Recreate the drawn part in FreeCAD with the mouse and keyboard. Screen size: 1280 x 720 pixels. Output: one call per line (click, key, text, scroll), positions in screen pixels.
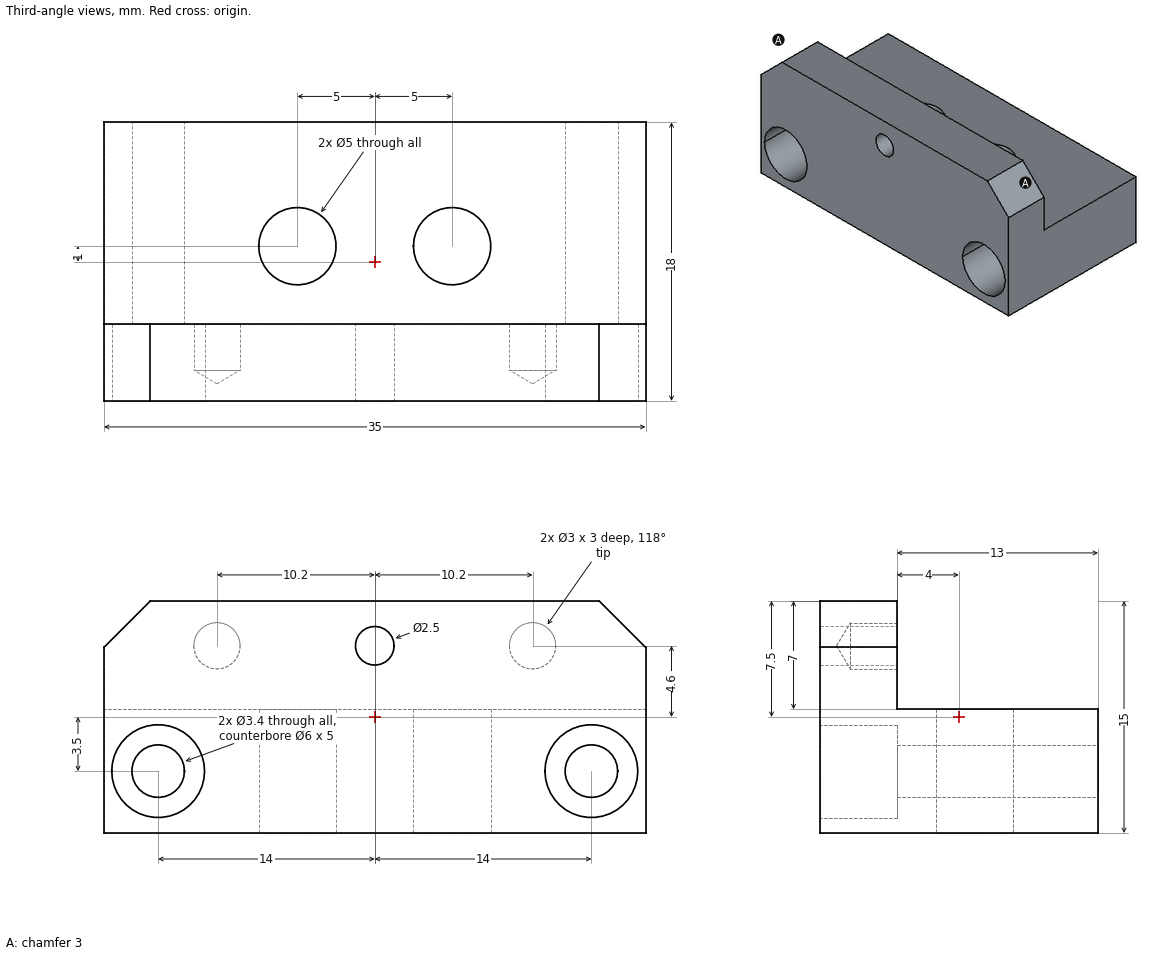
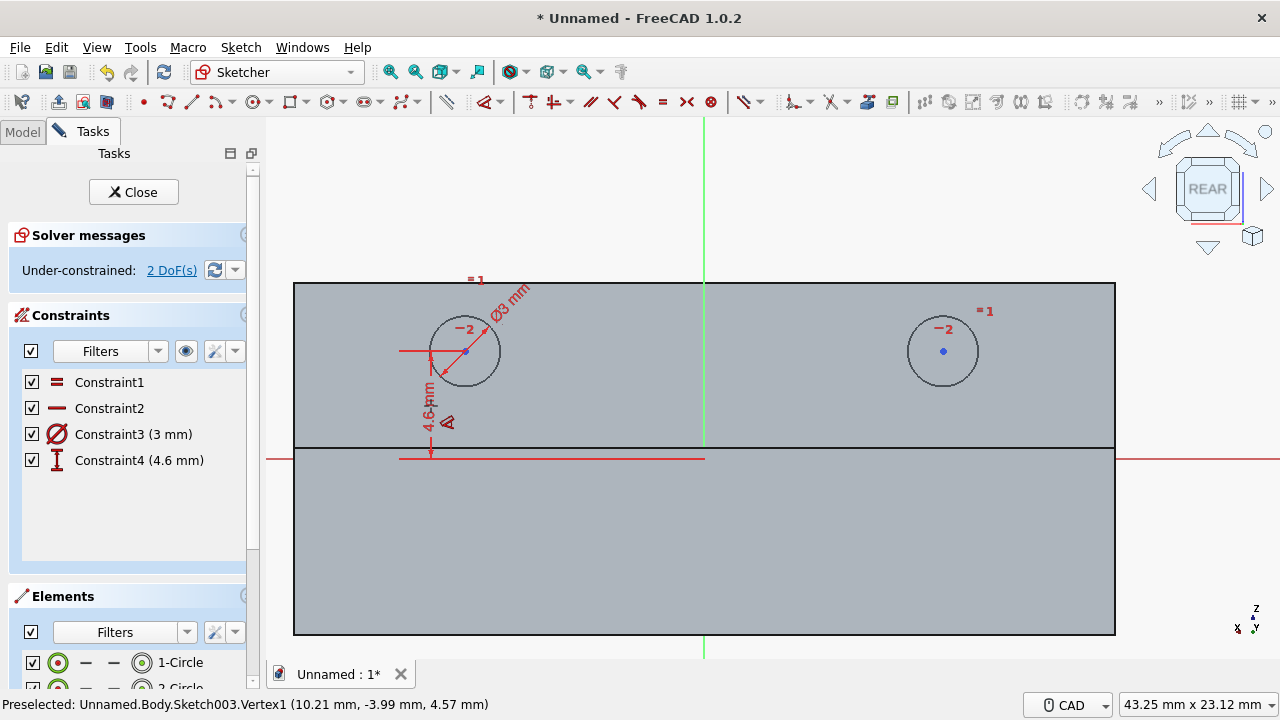
click(465, 351)
click(585, 493)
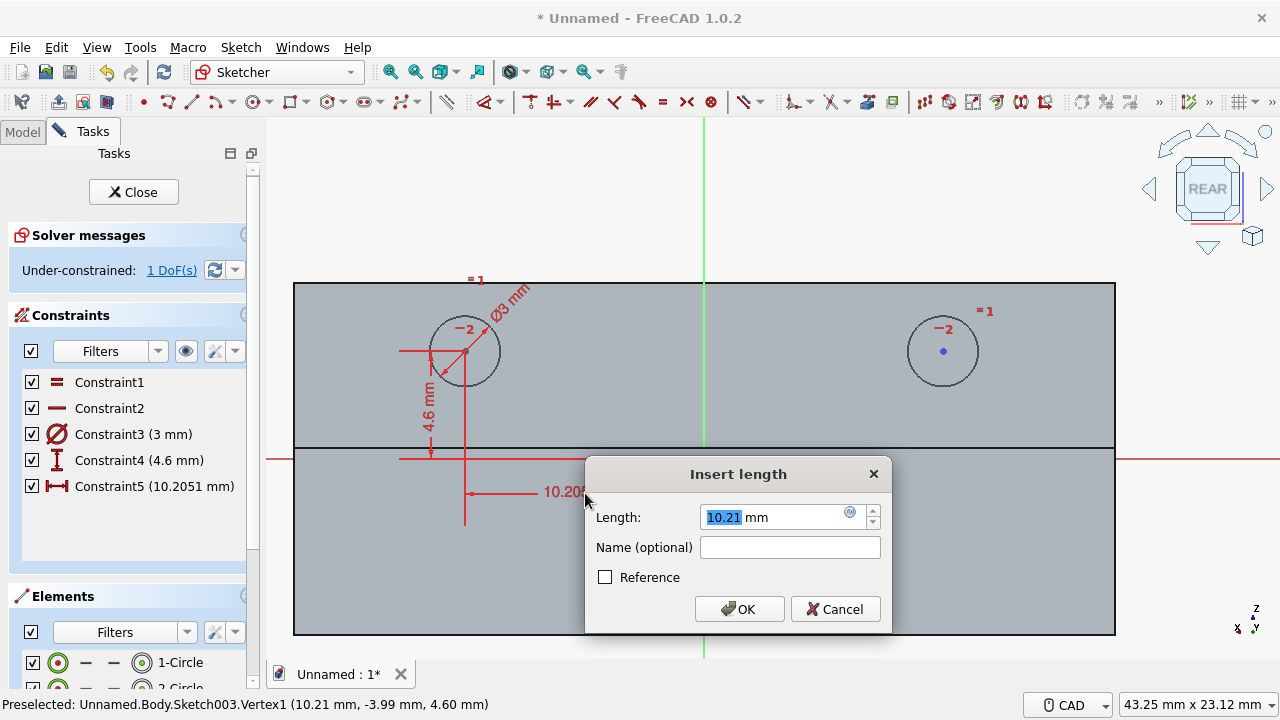
text(10.2)
key(Return)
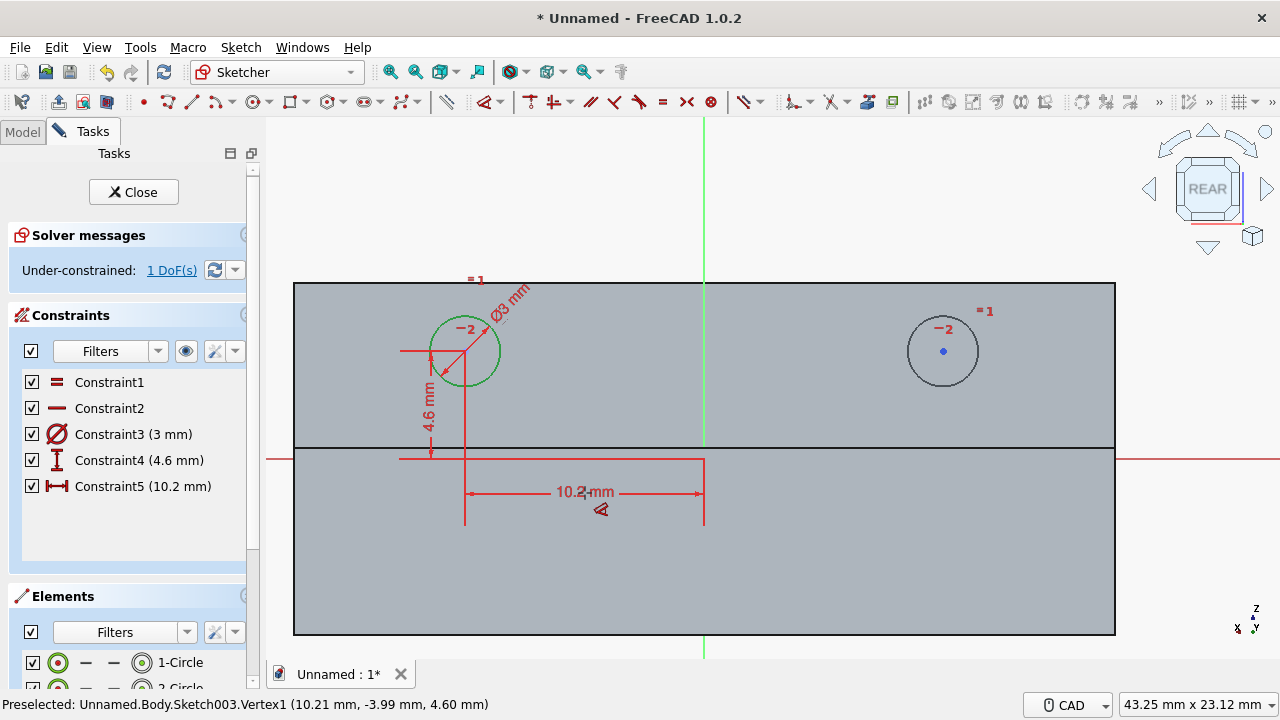
click(943, 351)
click(824, 493)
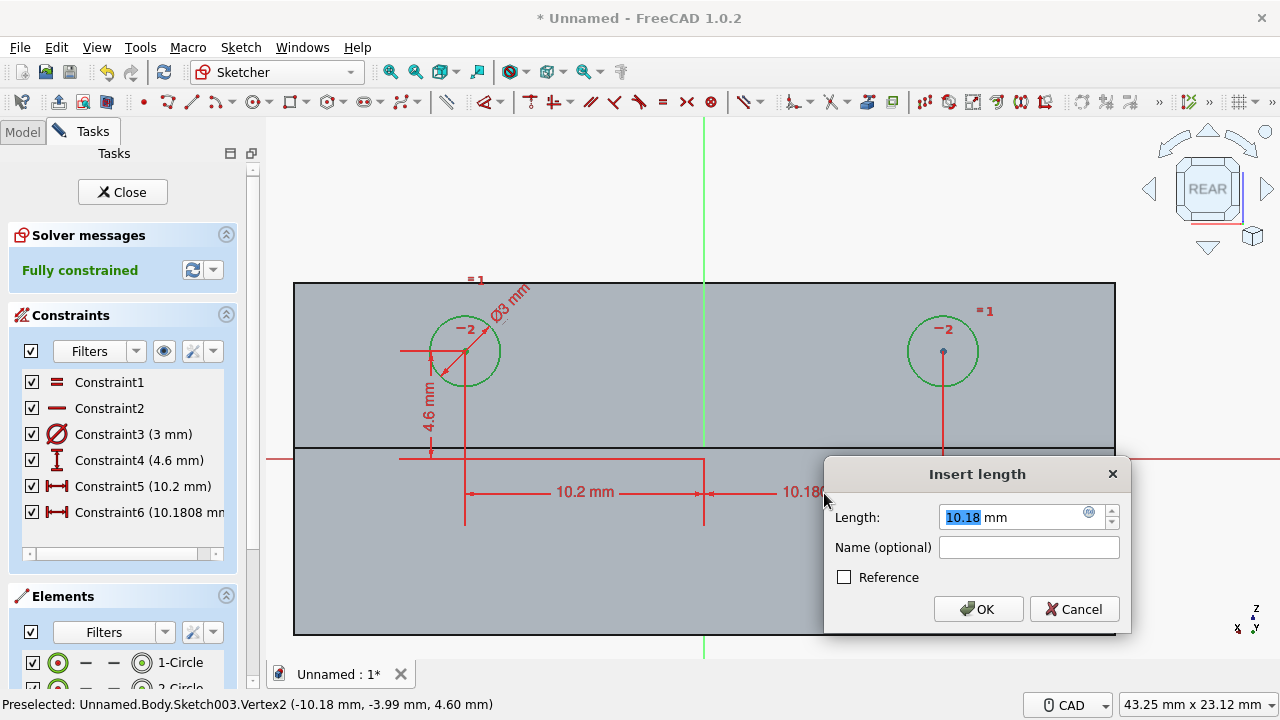
text(10.2)
key(Return)
key(Escape)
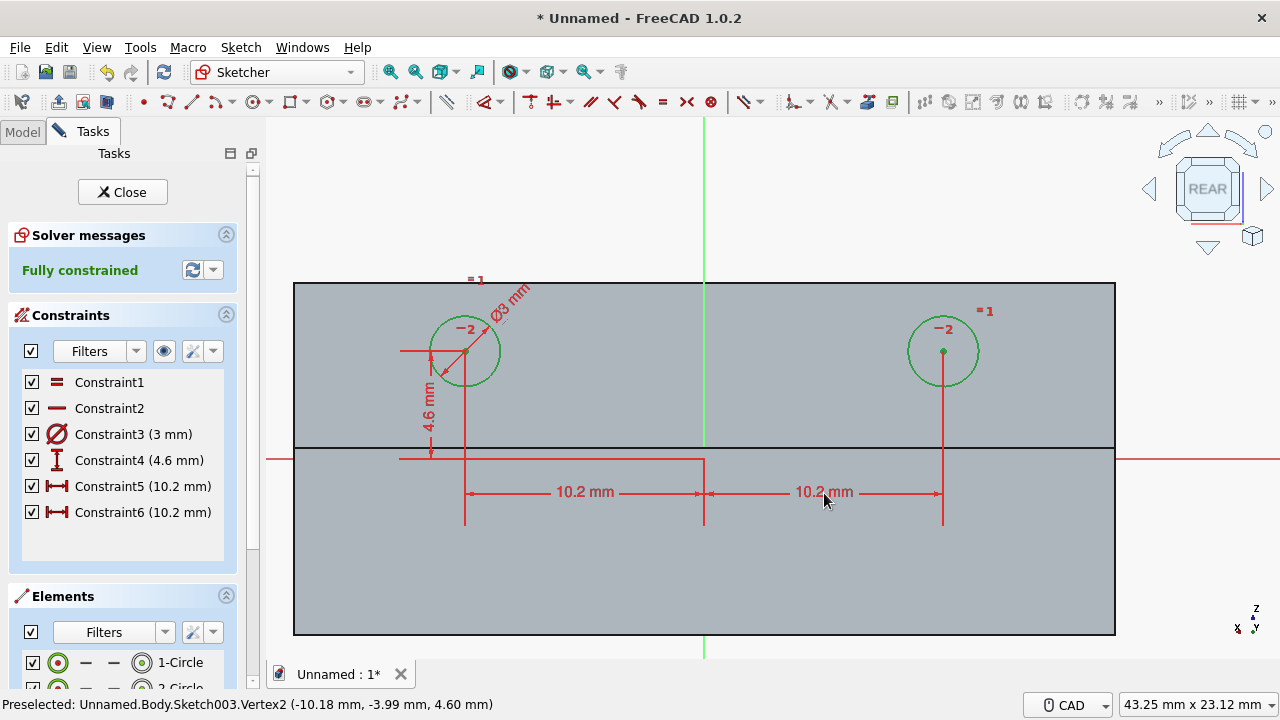
click(123, 192)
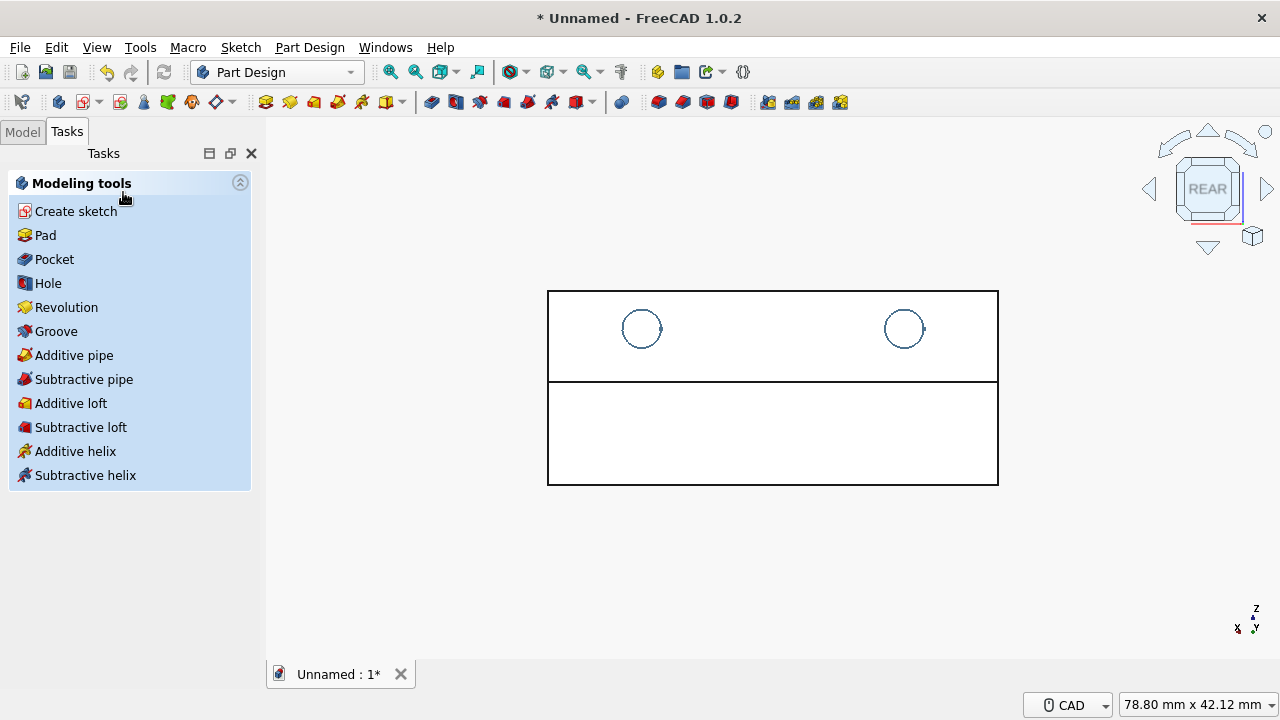
click(456, 102)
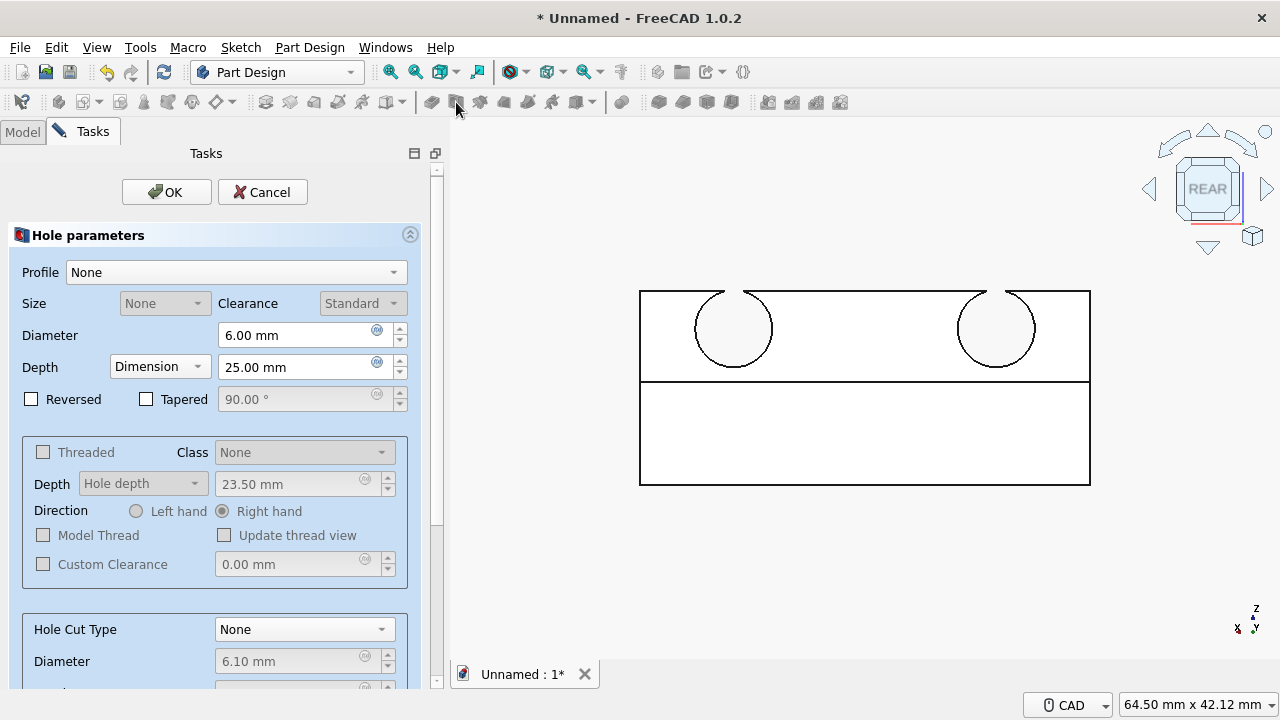
triple_click(305, 335)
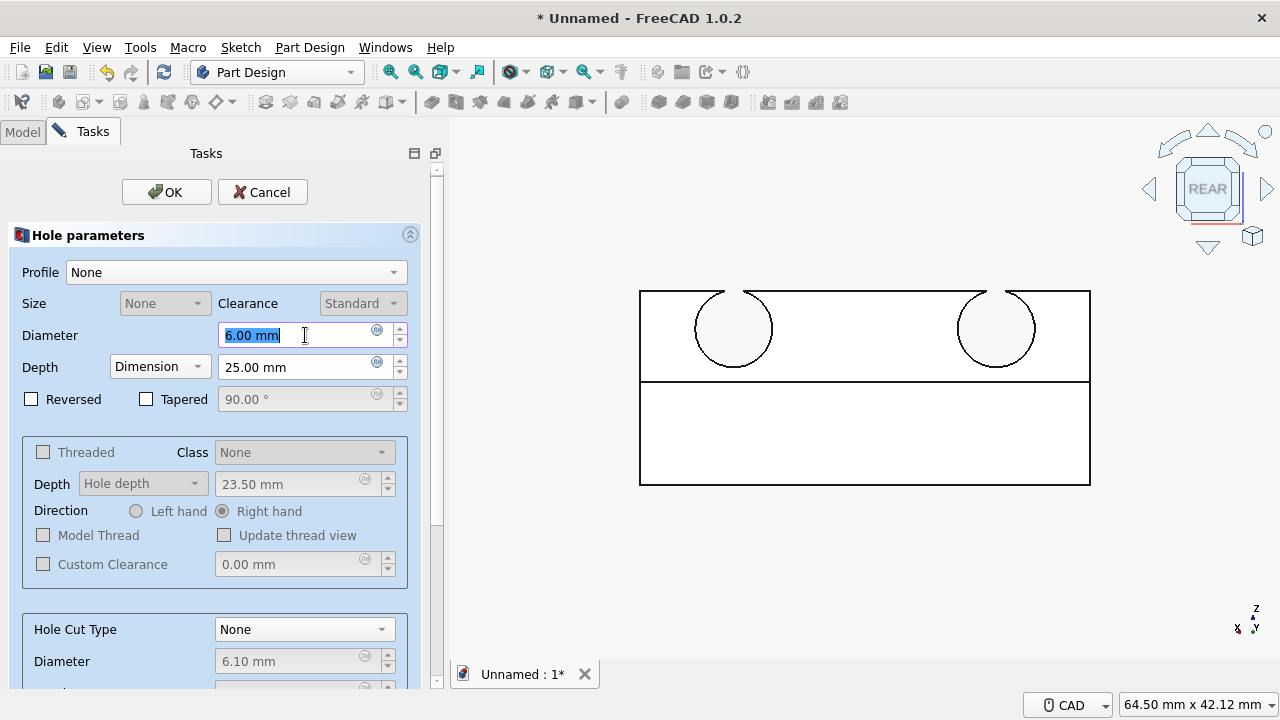
text(3)
key(Tab)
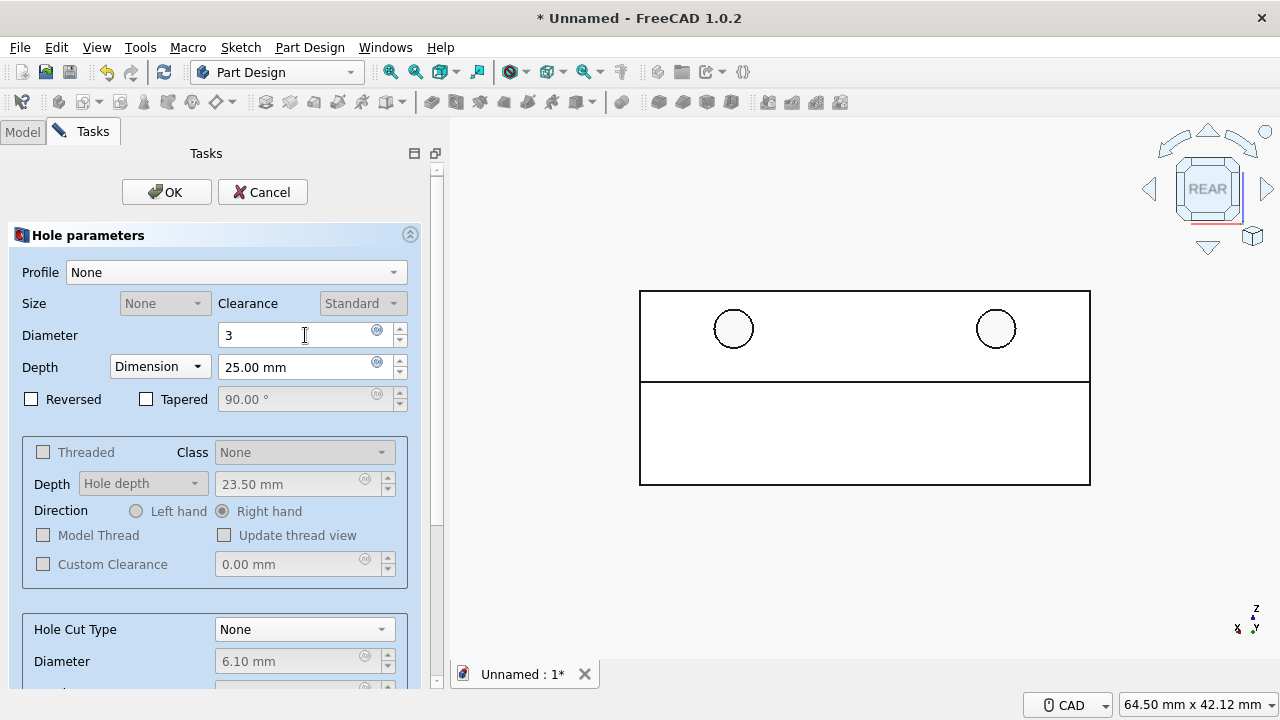
triple_click(305, 367)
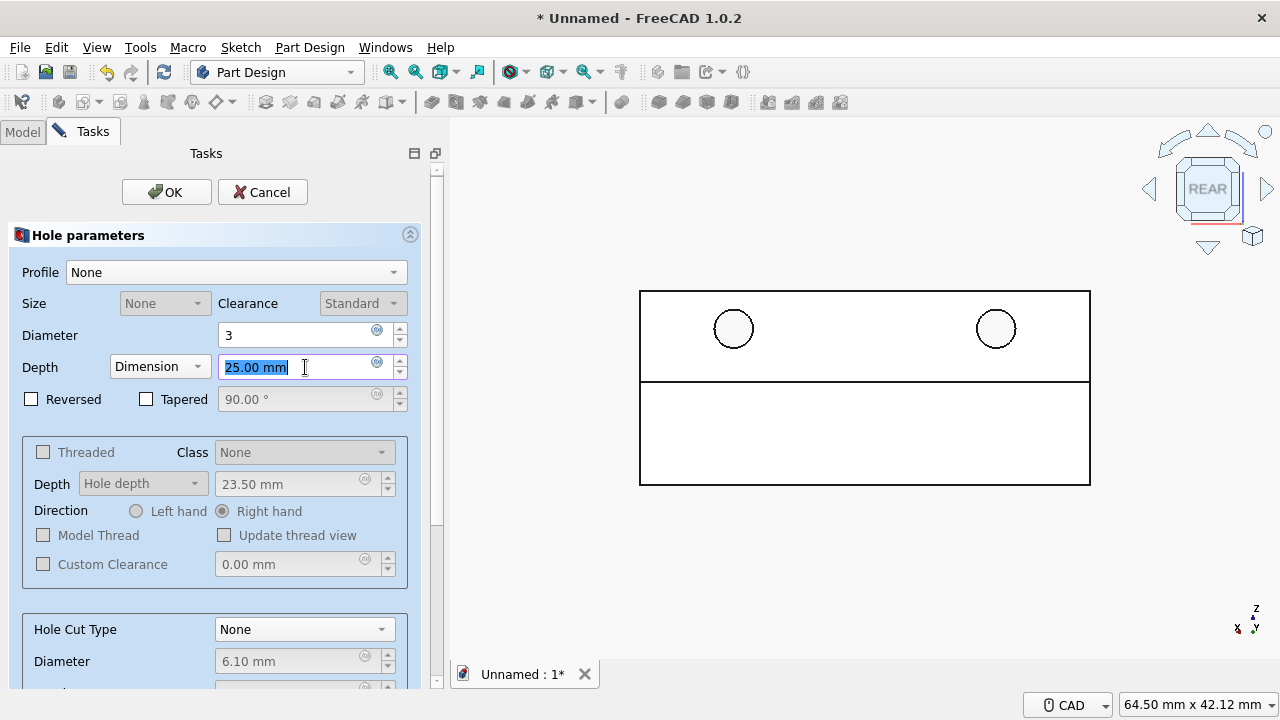
text(3)
key(Tab)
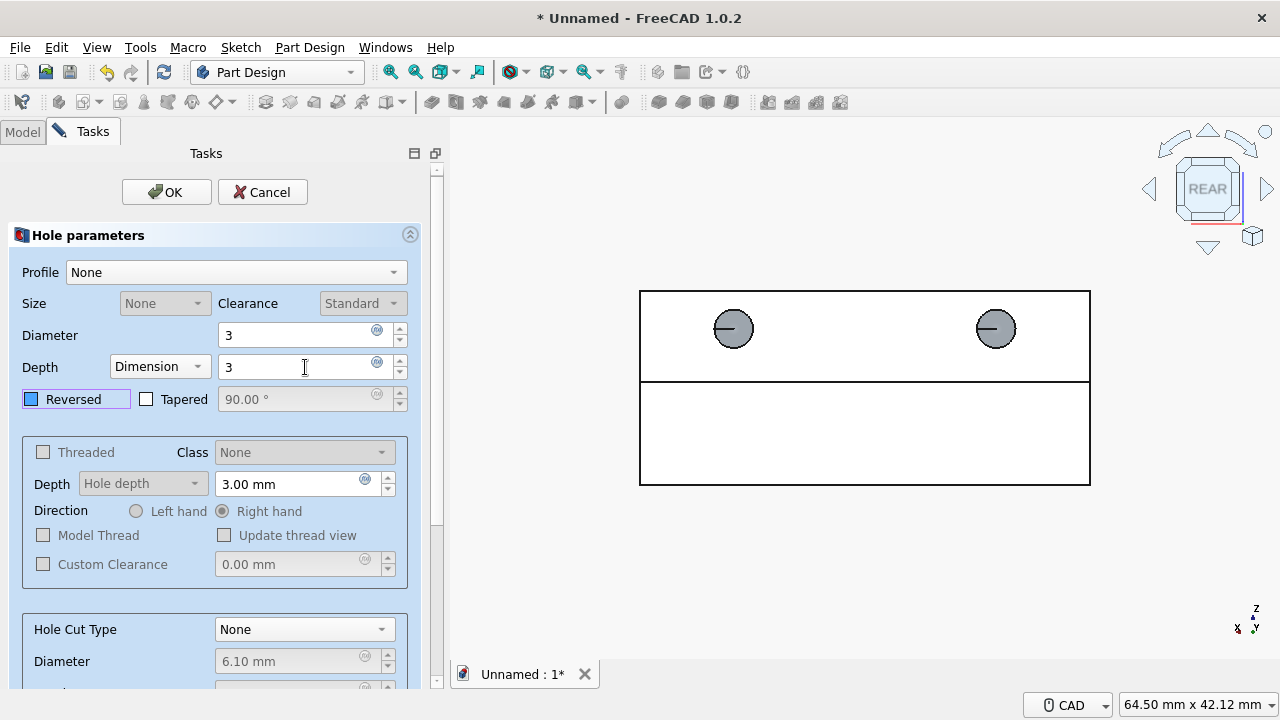
click(167, 192)